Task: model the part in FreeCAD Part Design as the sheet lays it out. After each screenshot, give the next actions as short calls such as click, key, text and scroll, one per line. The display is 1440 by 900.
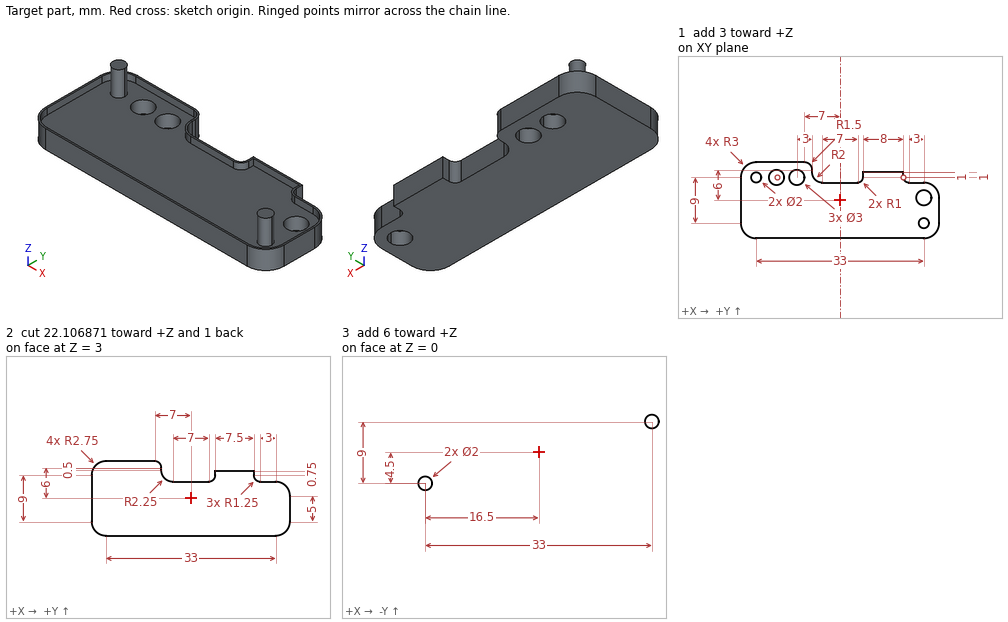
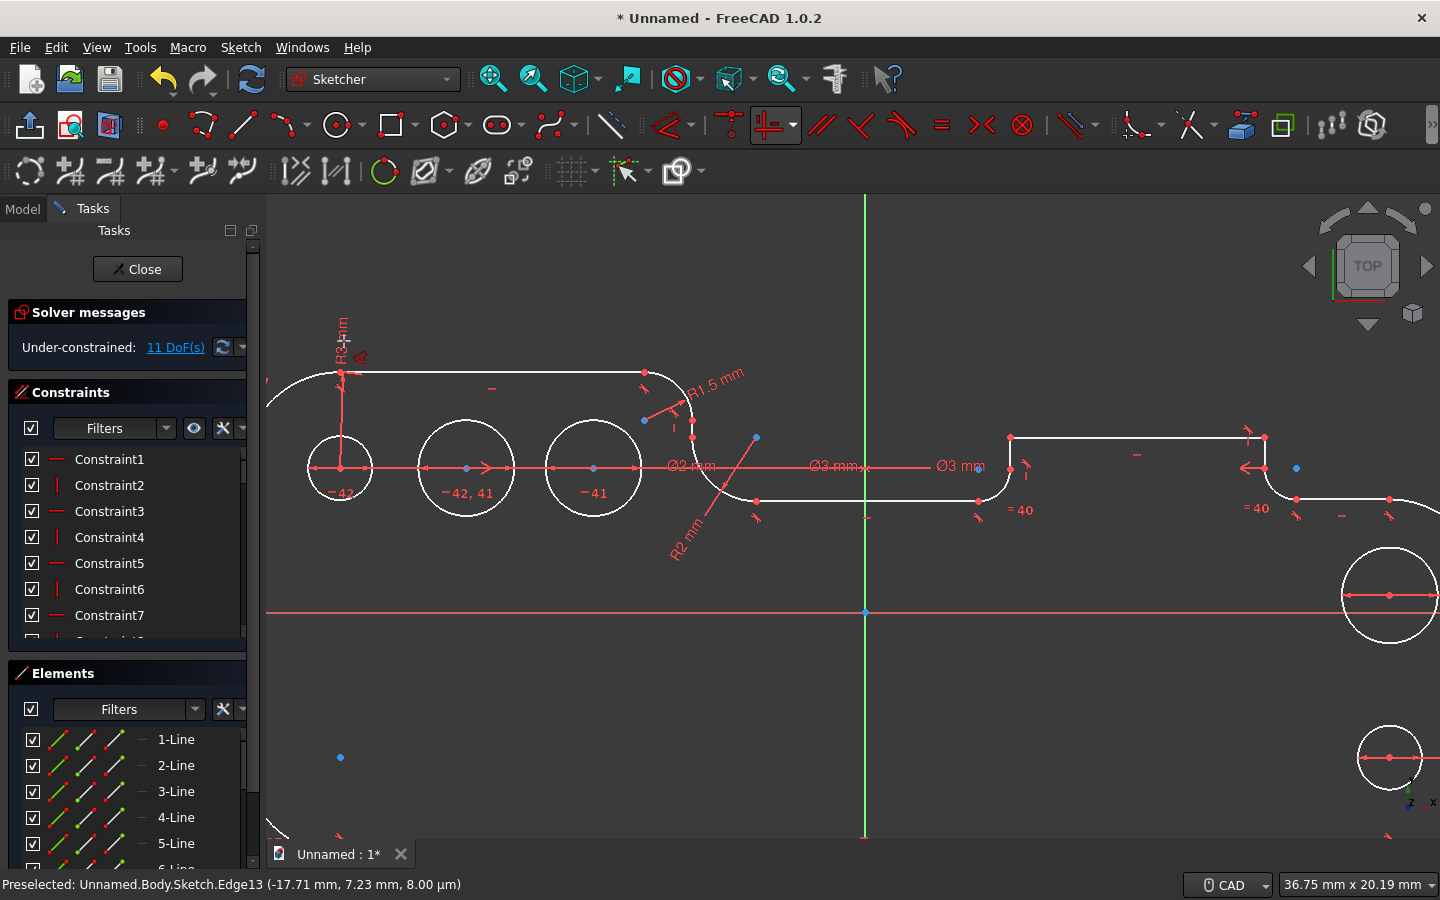
scroll(1268, 482, up, 2)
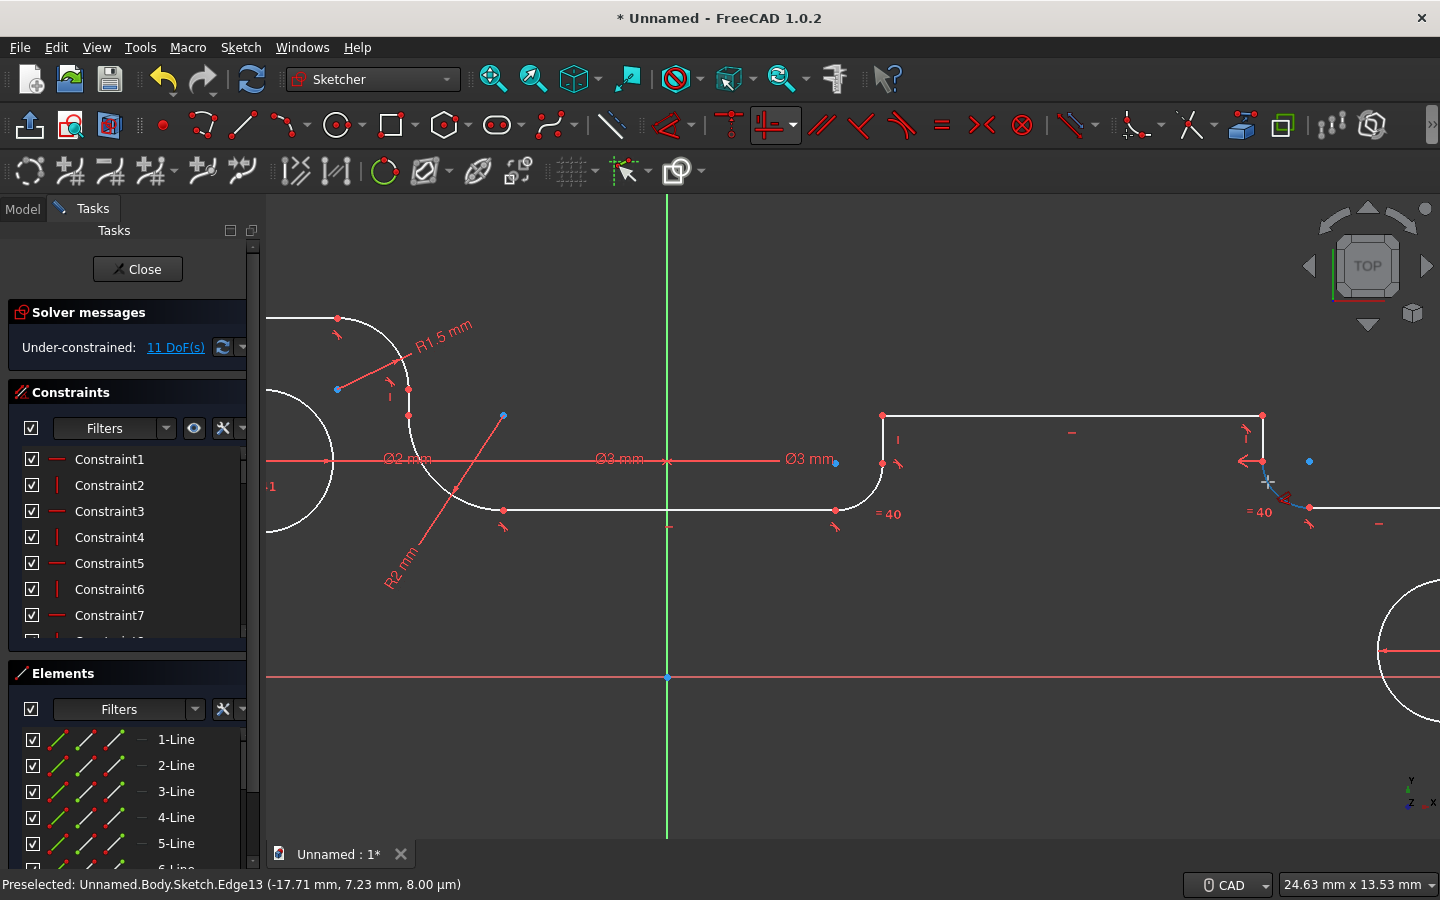
click(1268, 482)
click(1239, 496)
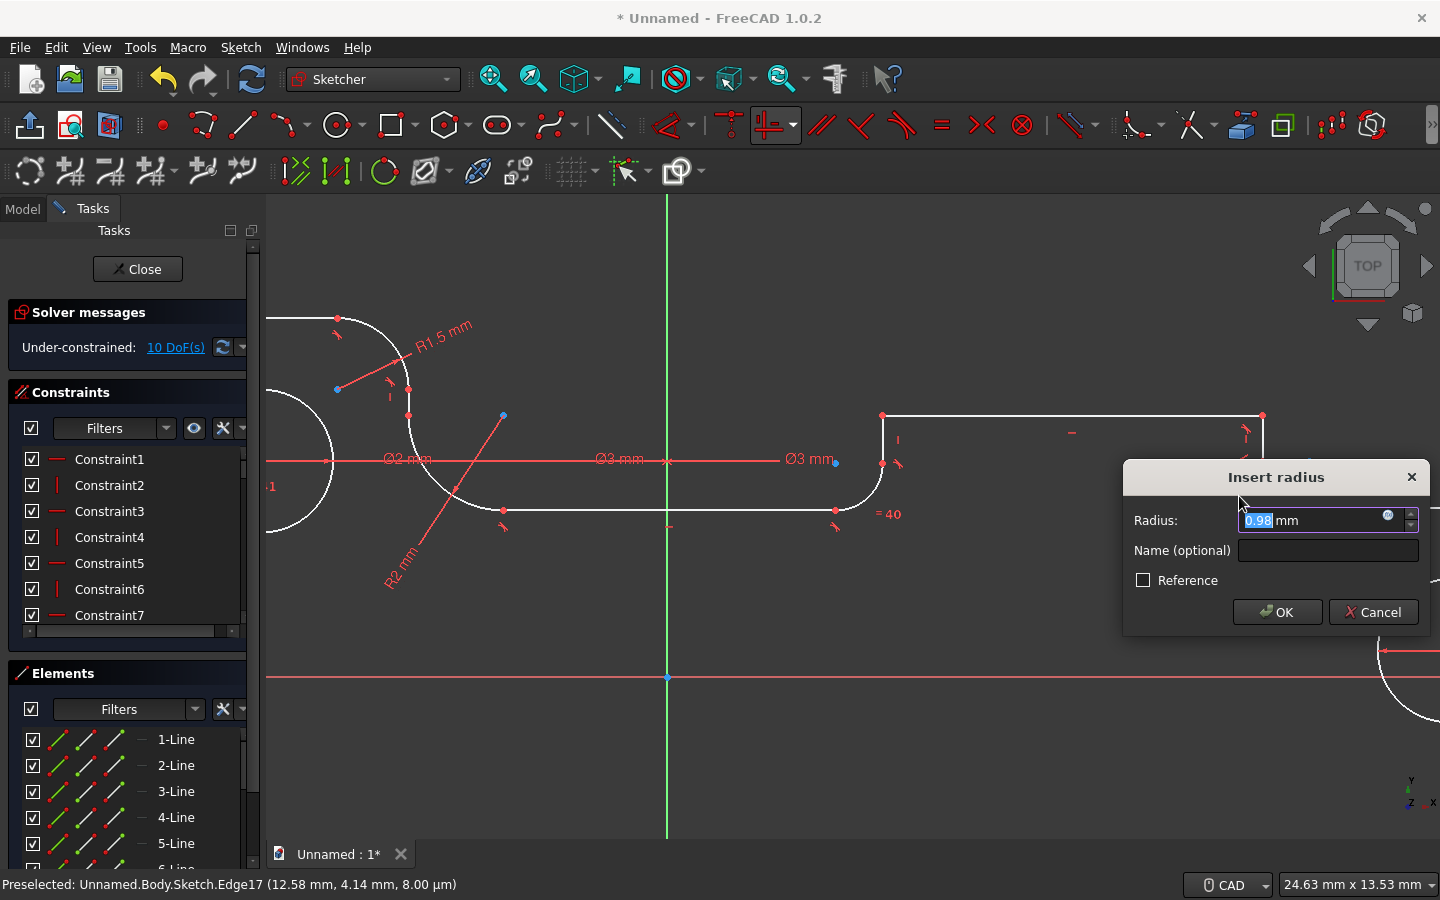
text(1)
key(Return)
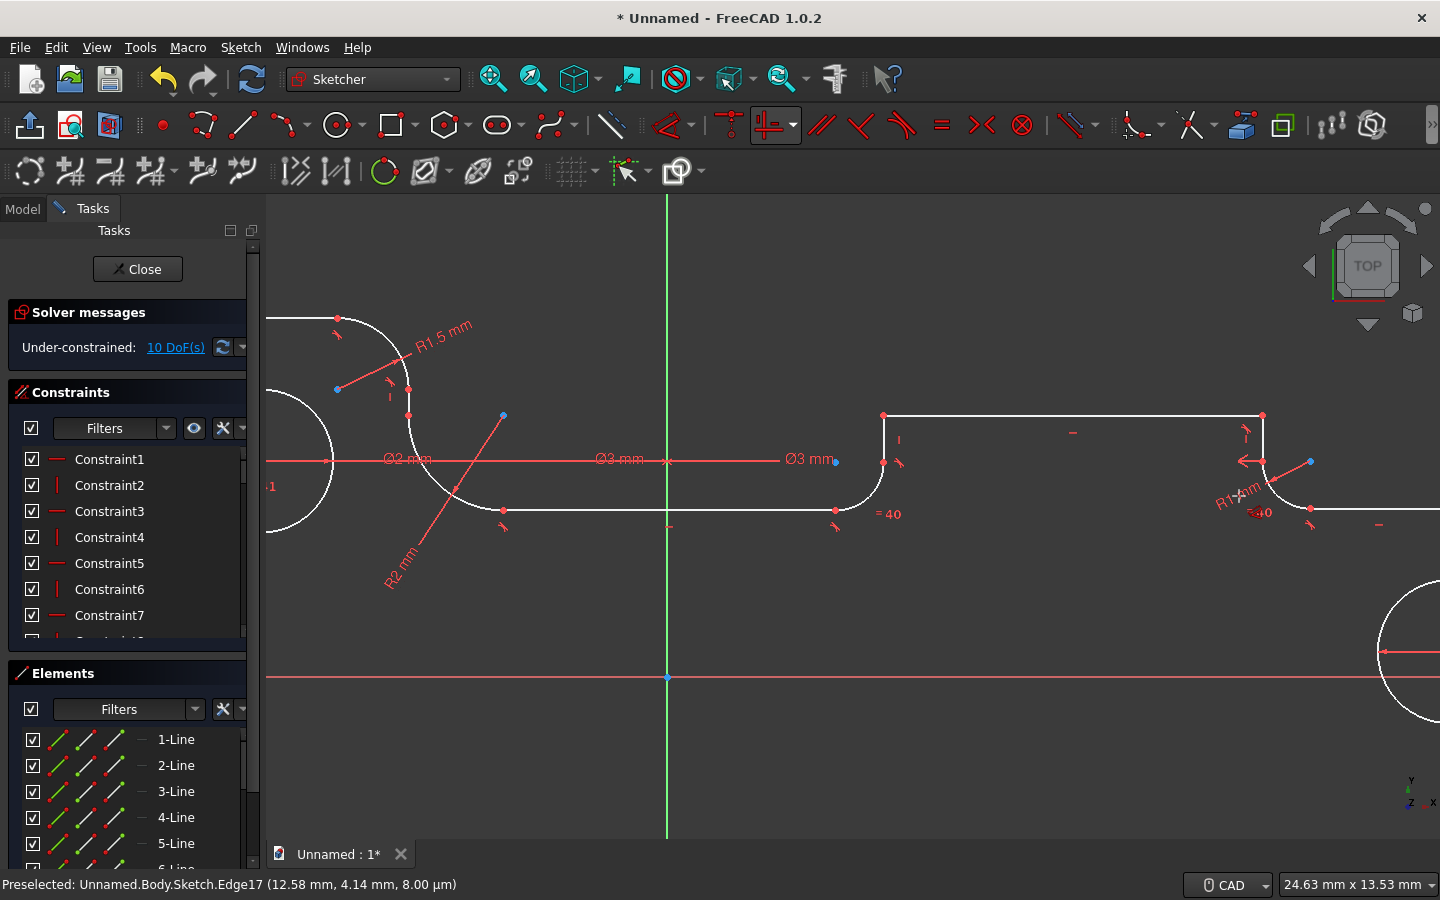
click(736, 510)
click(594, 476)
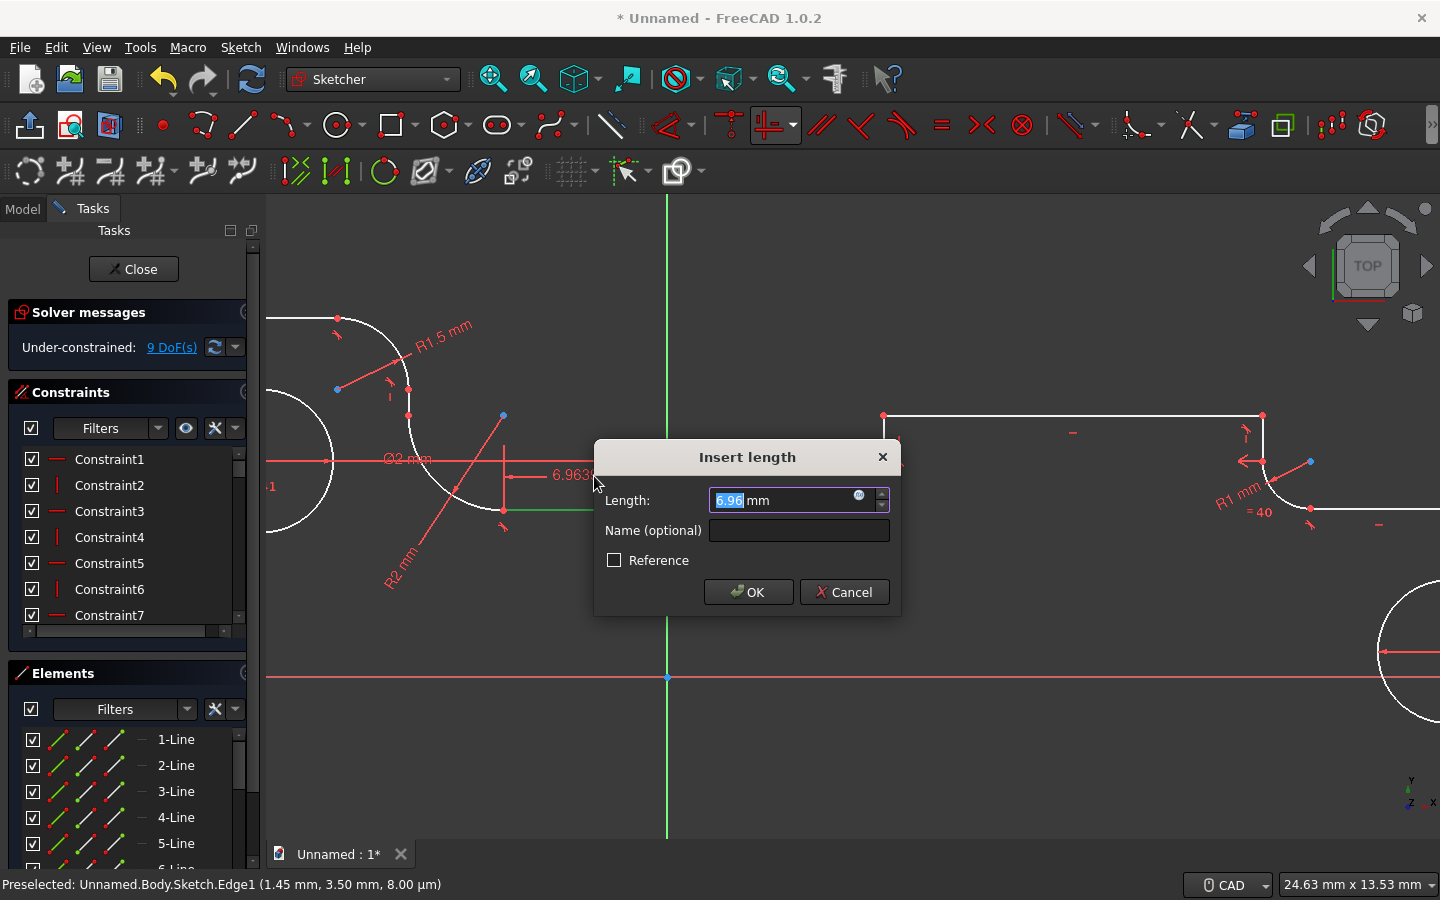
text(7)
key(Return)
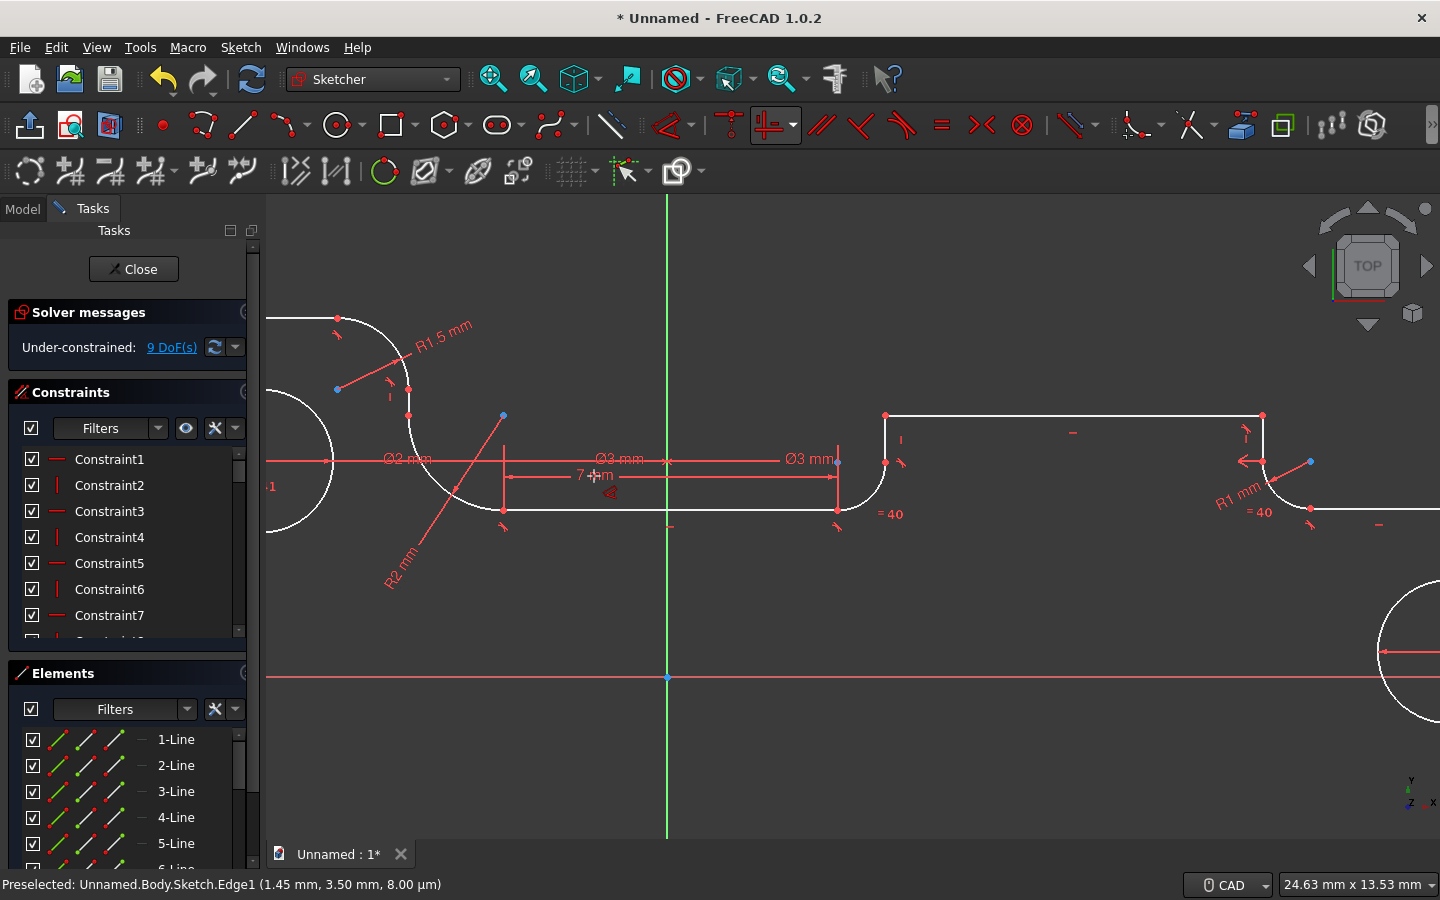
scroll(853, 423, down, 5)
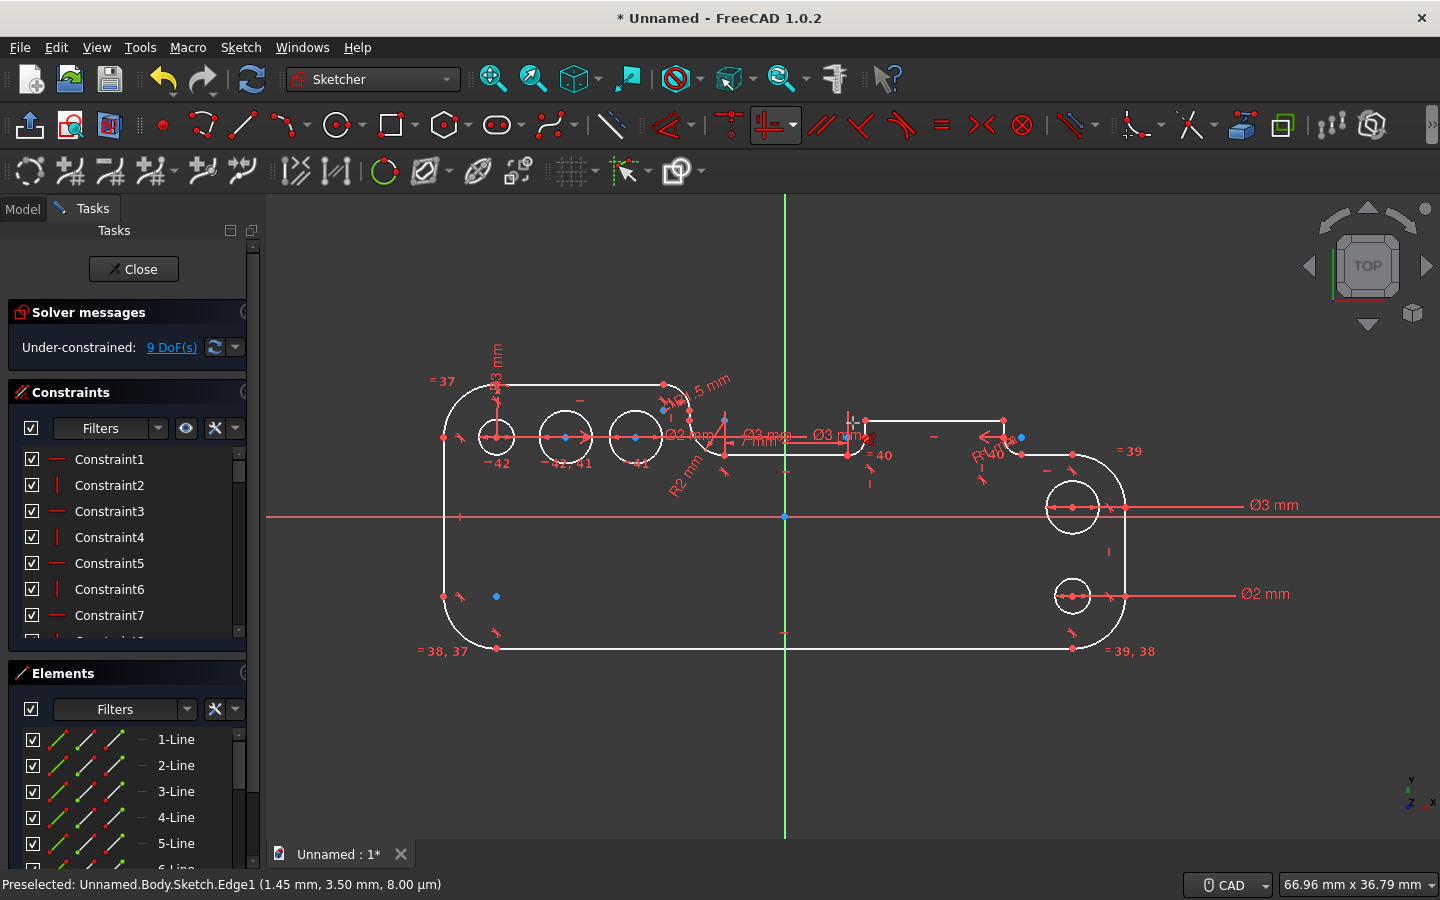
click(444, 485)
click(410, 480)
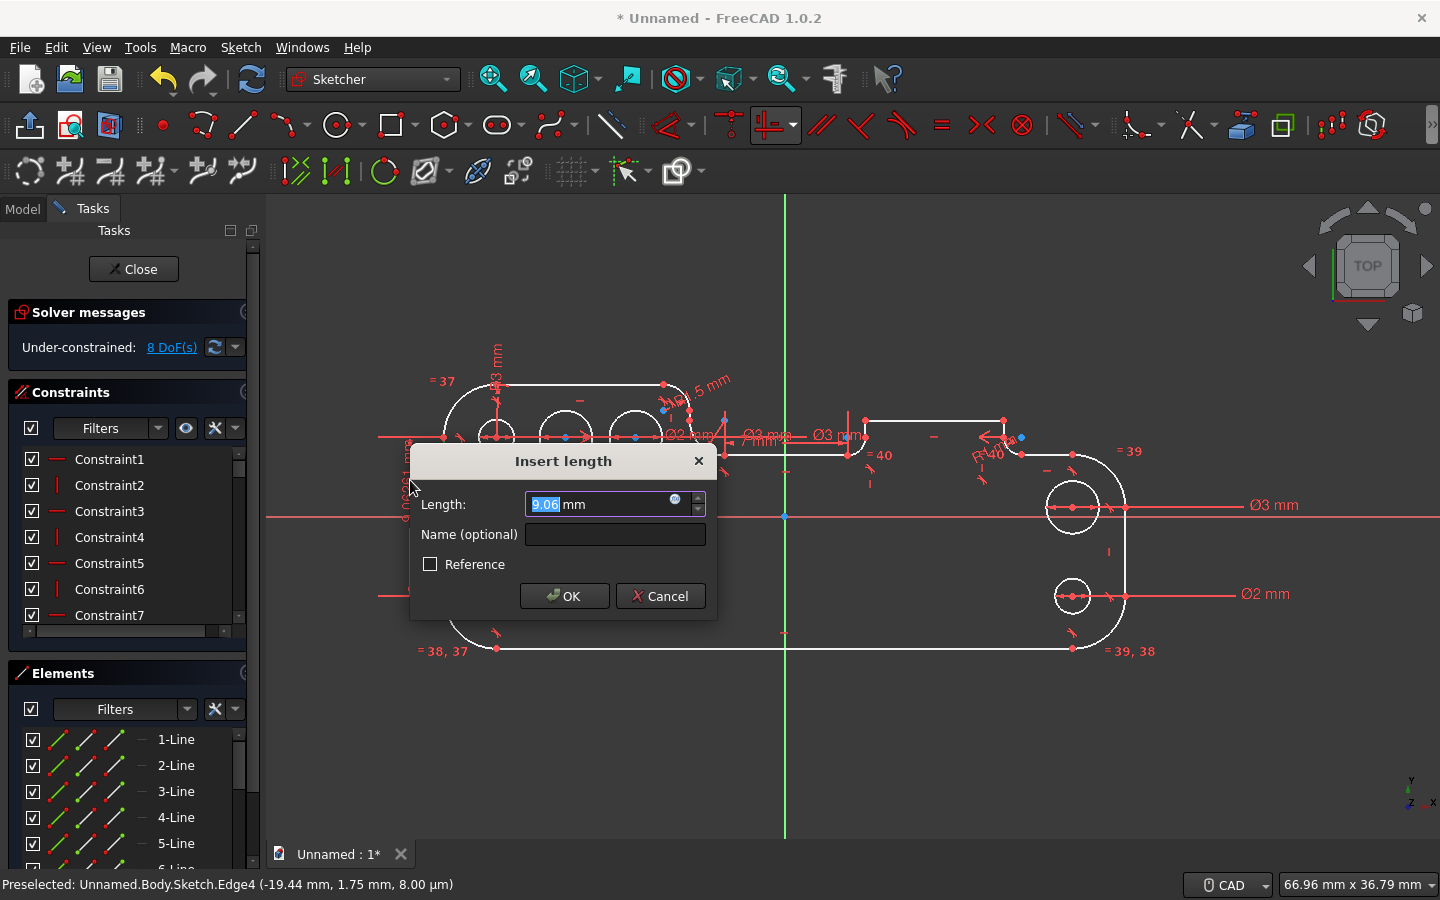
text(9)
key(Return)